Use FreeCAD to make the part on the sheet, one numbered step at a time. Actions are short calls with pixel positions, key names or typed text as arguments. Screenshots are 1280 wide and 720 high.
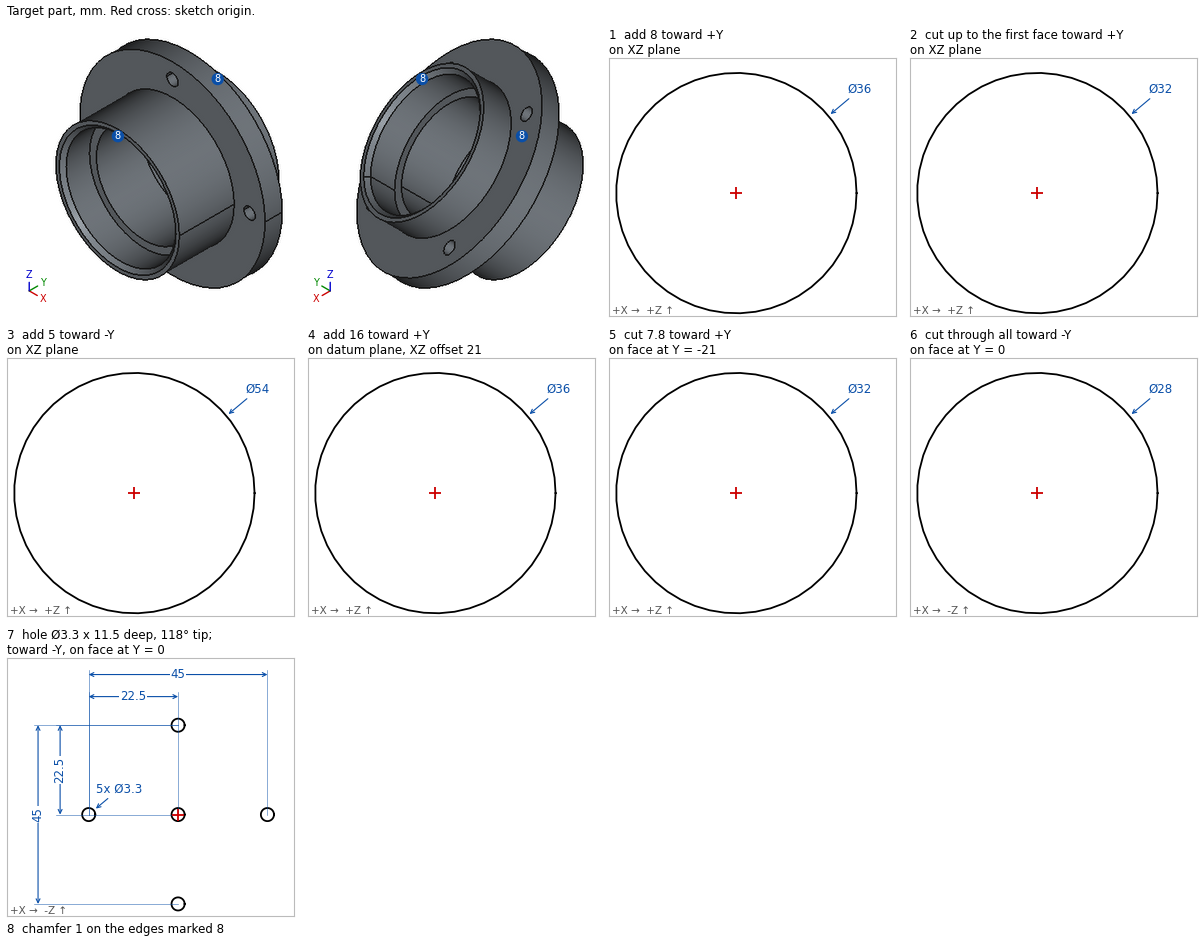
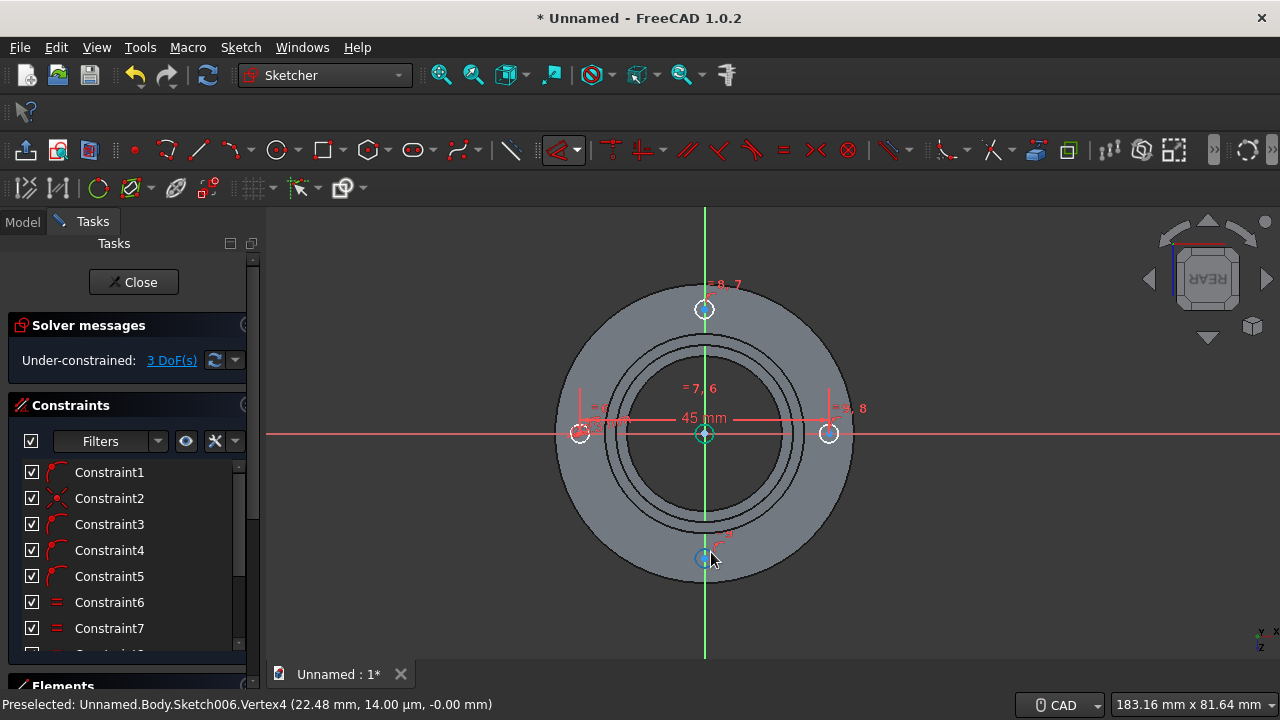
click(705, 310)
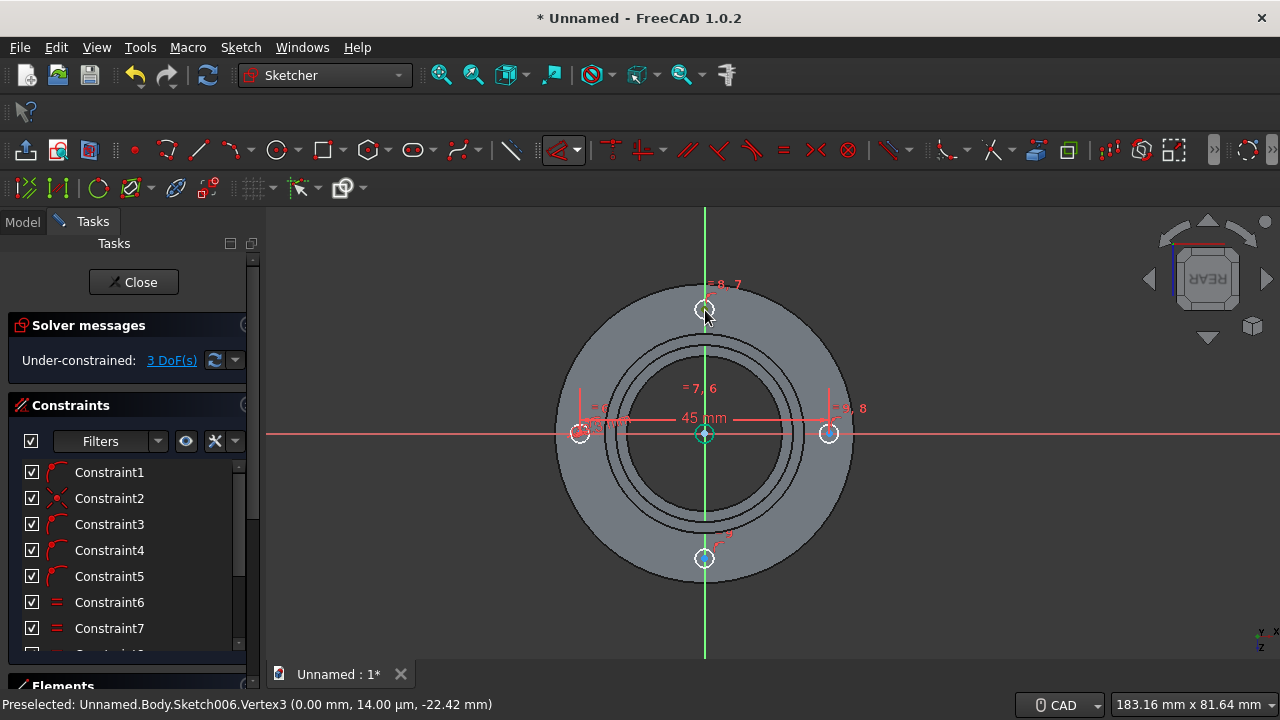
click(705, 558)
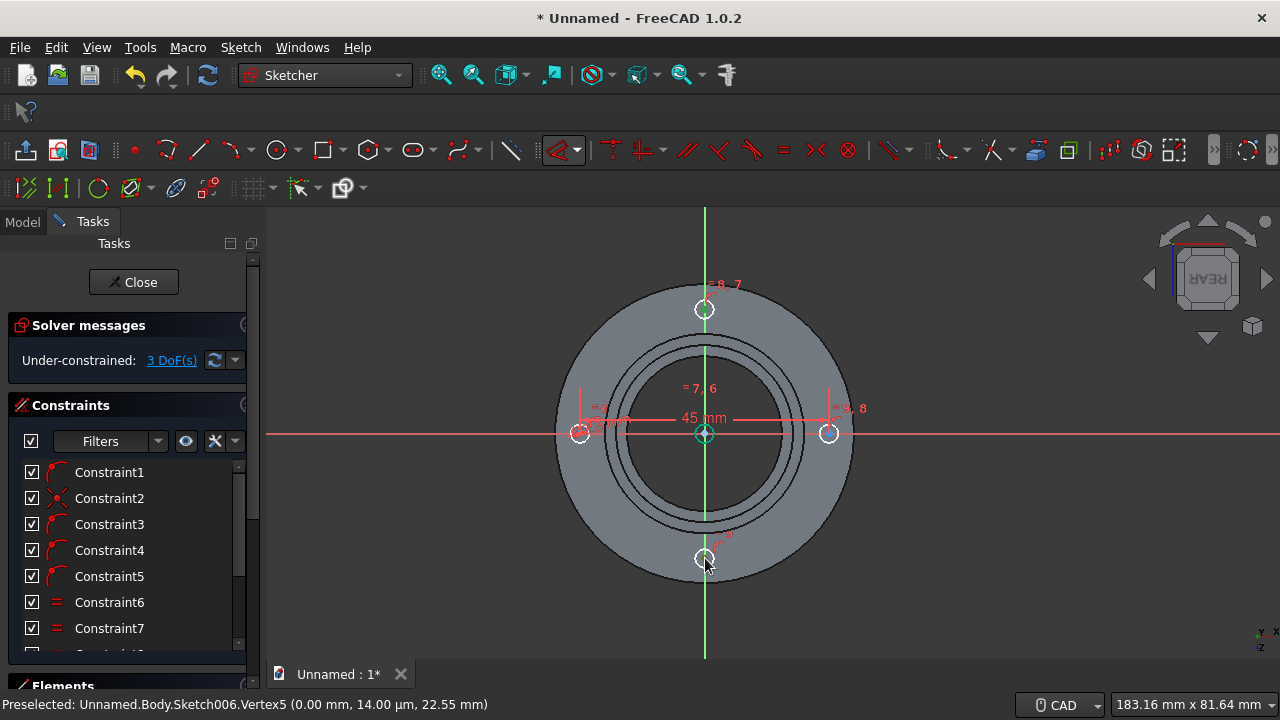
click(580, 150)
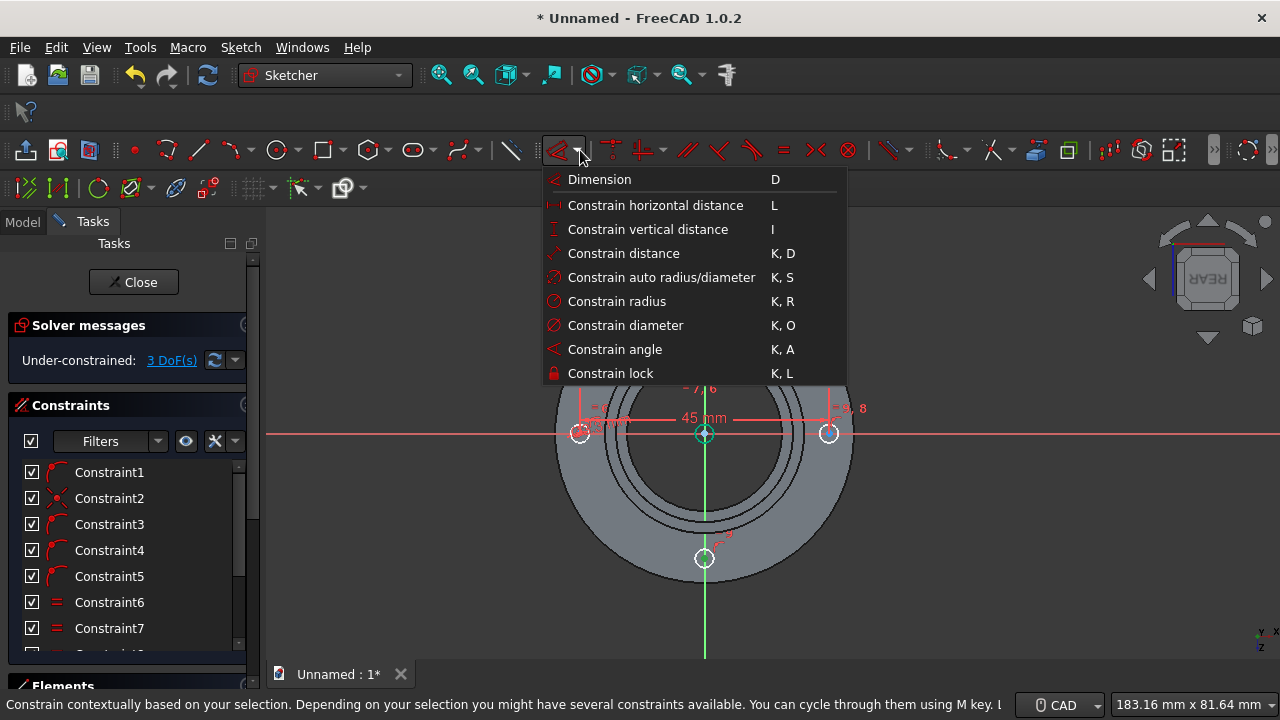
click(695, 229)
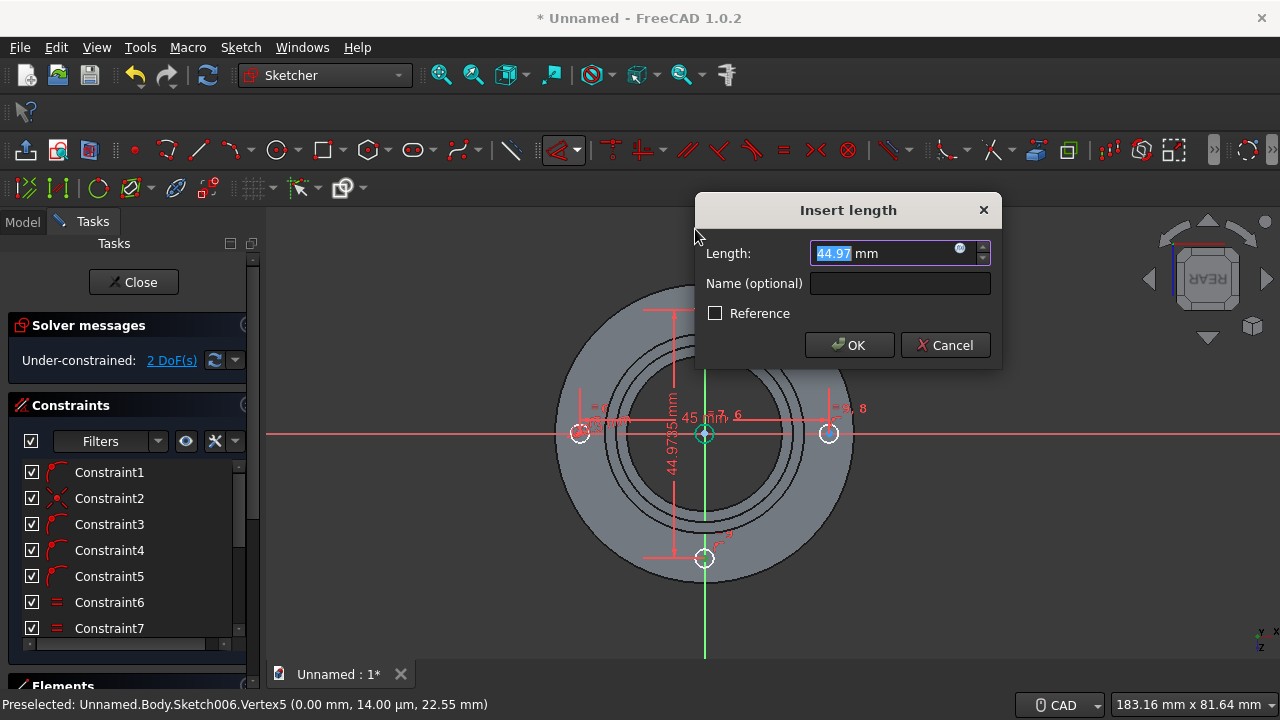
text(45)
key(Return)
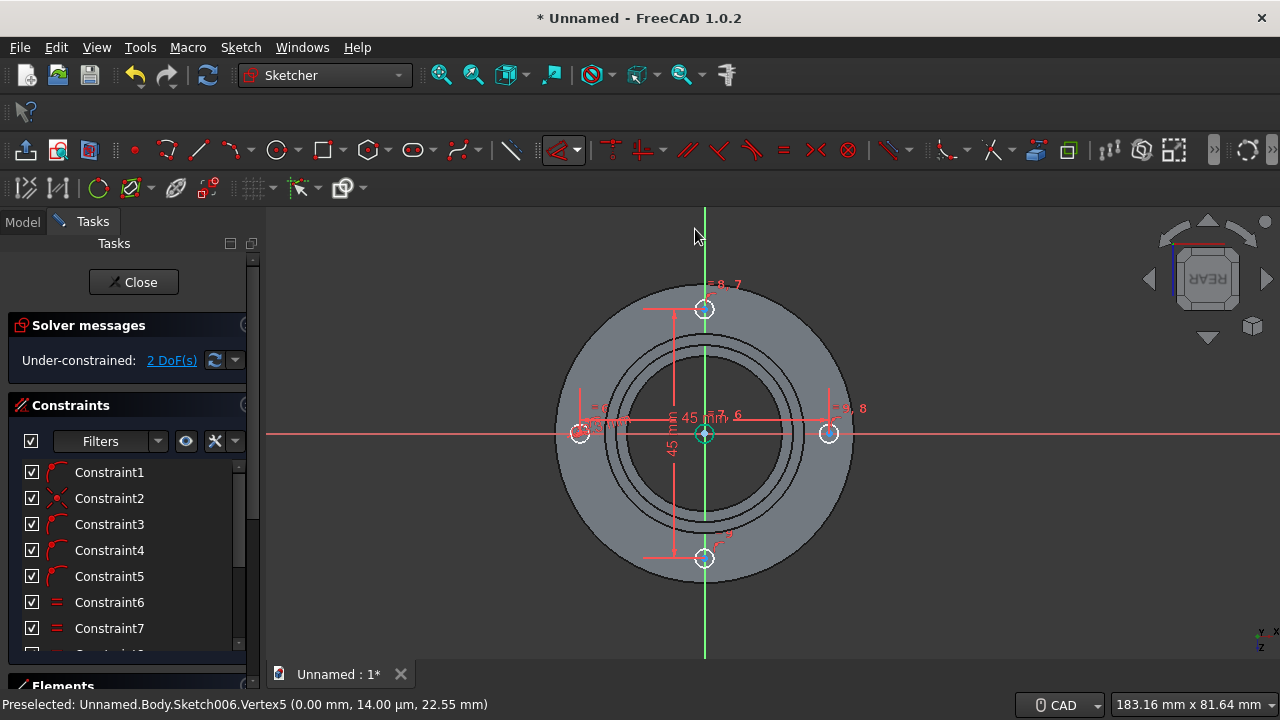
click(580, 434)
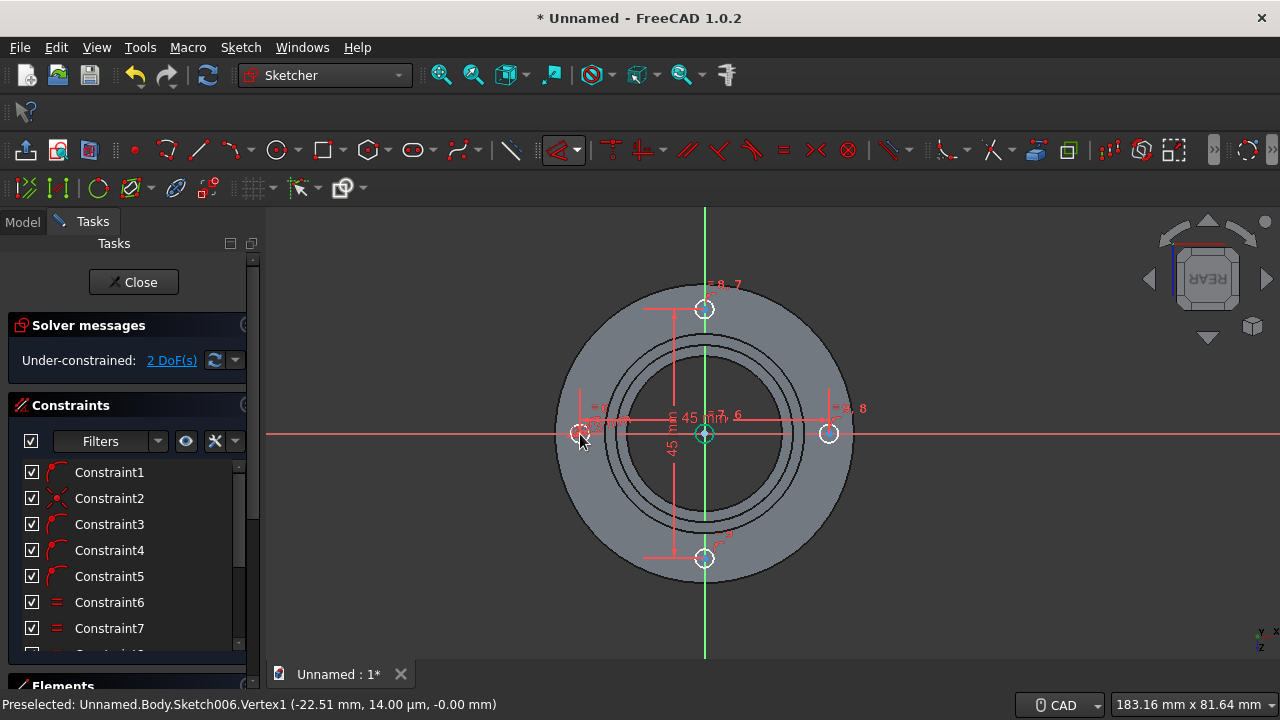
click(580, 150)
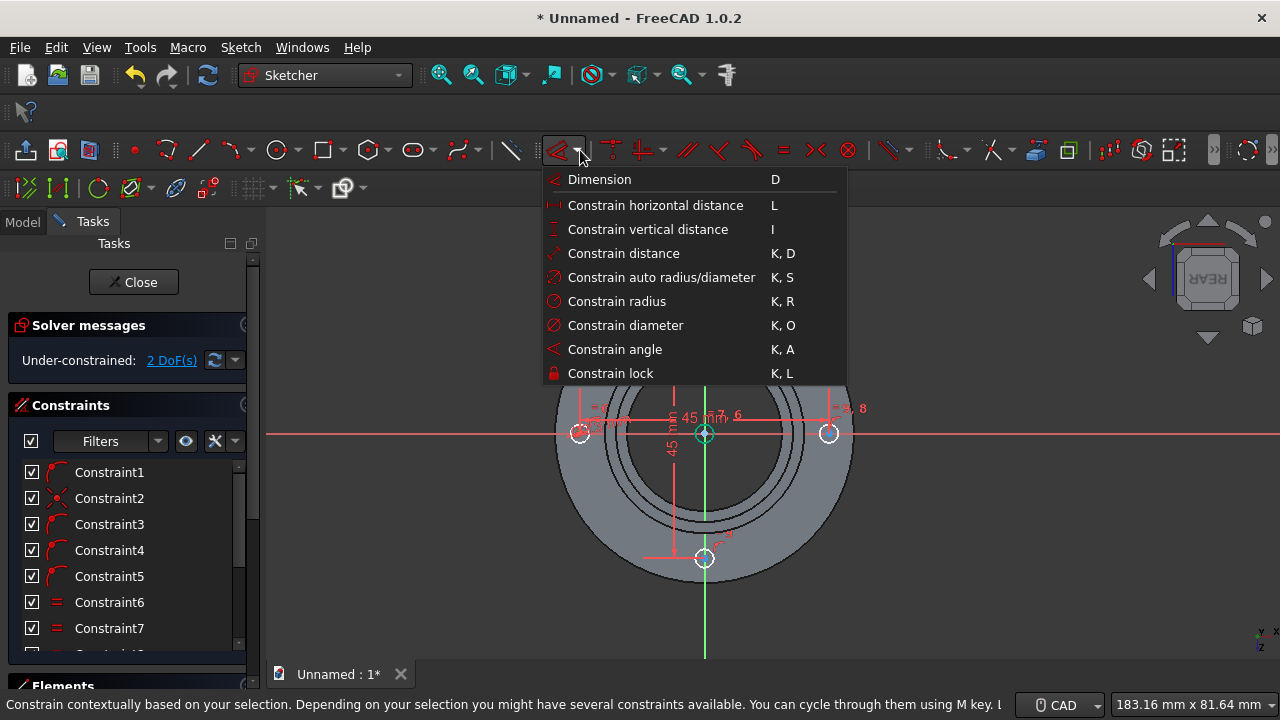
click(695, 205)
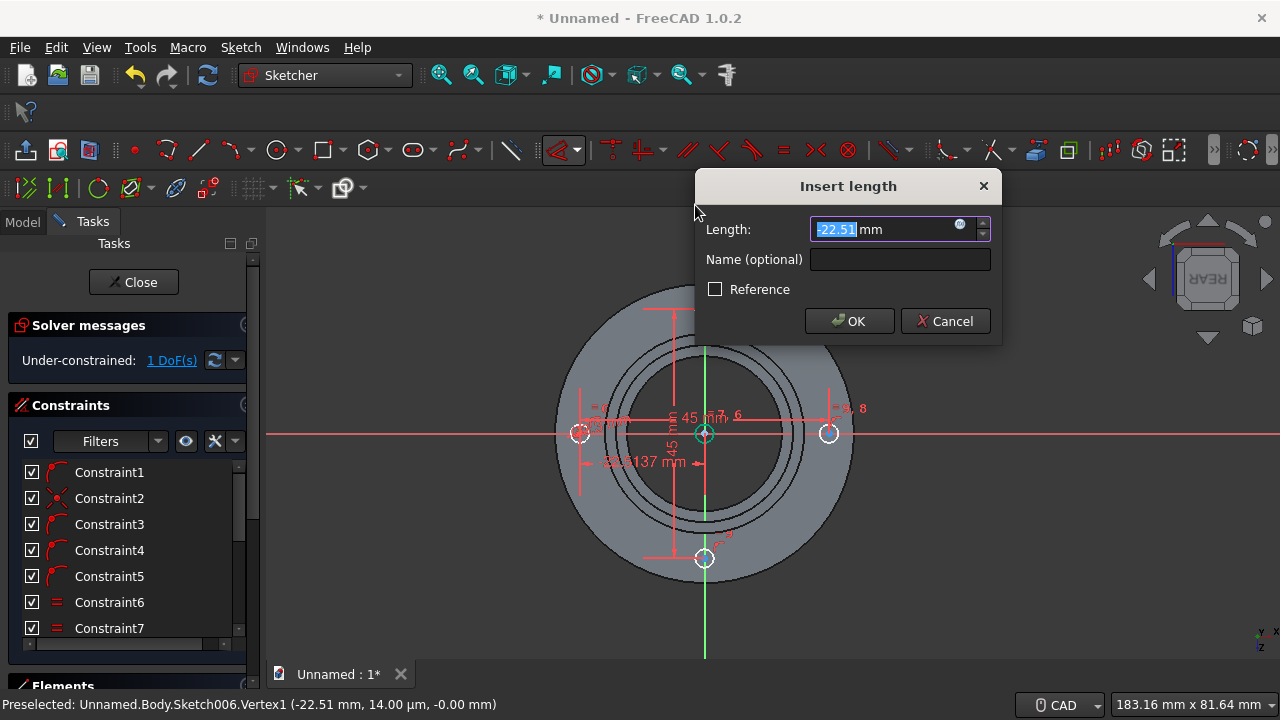
text(-22.5)
key(Return)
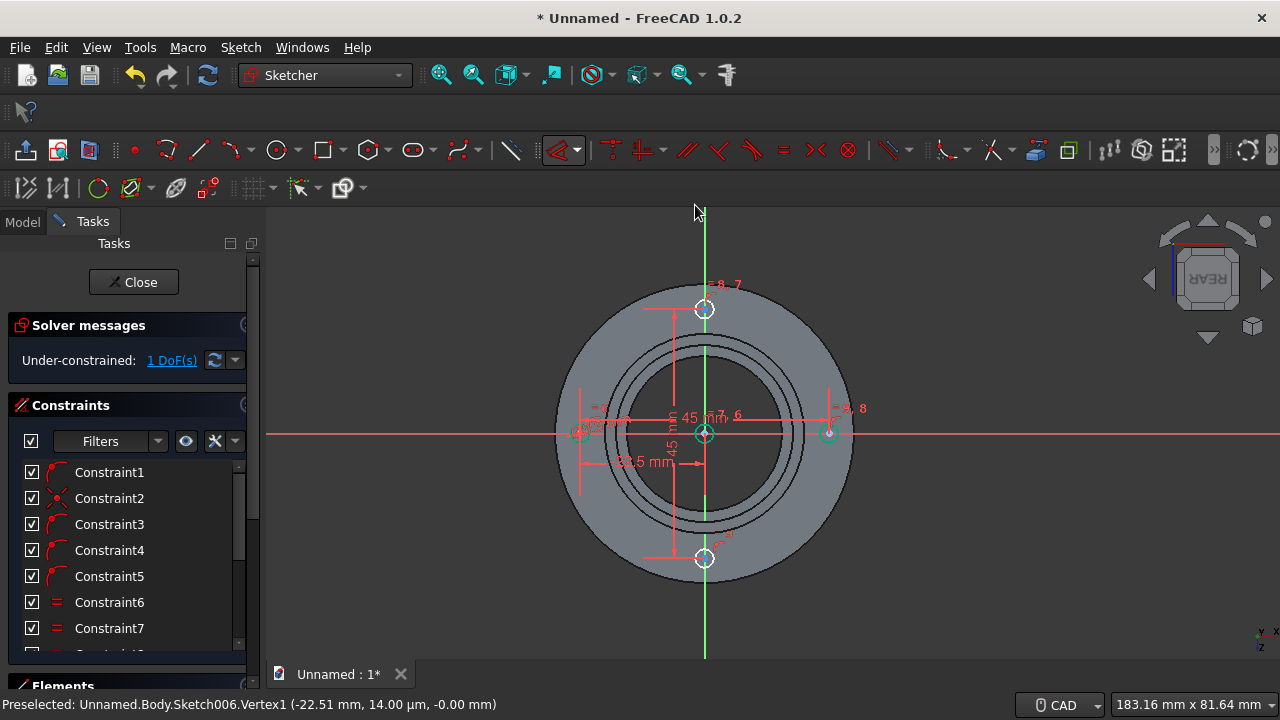
click(705, 309)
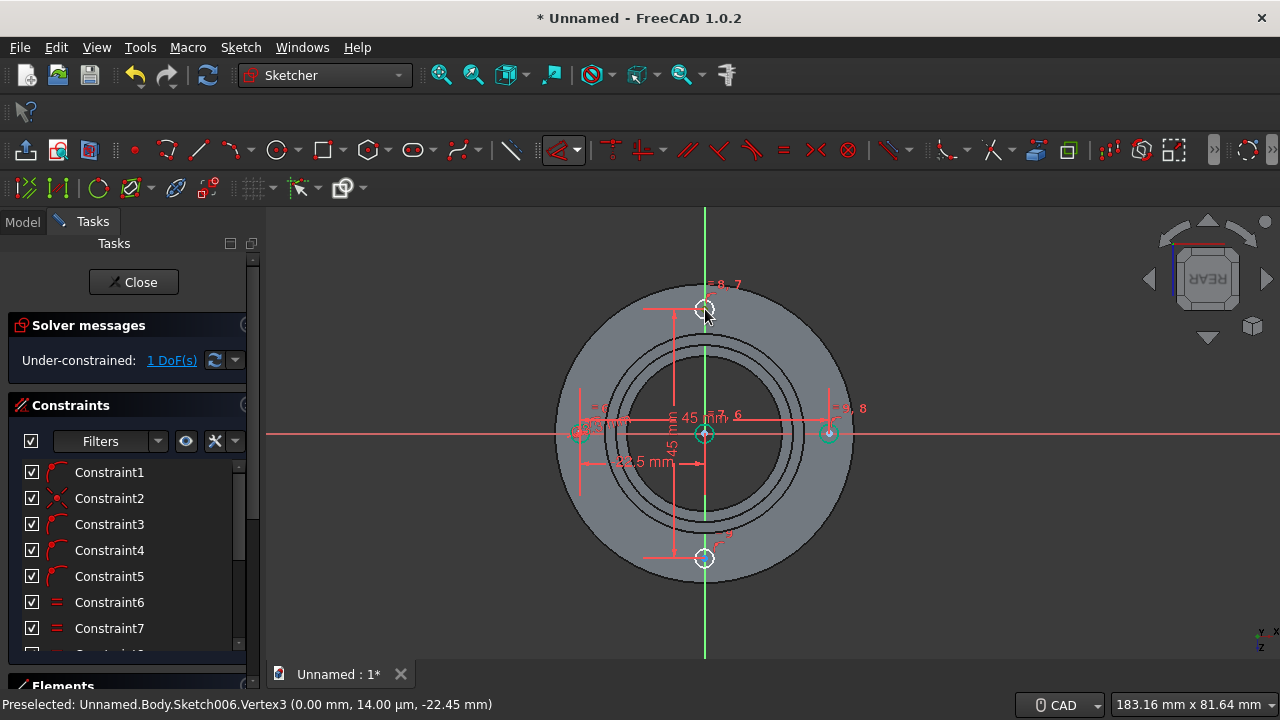
click(580, 150)